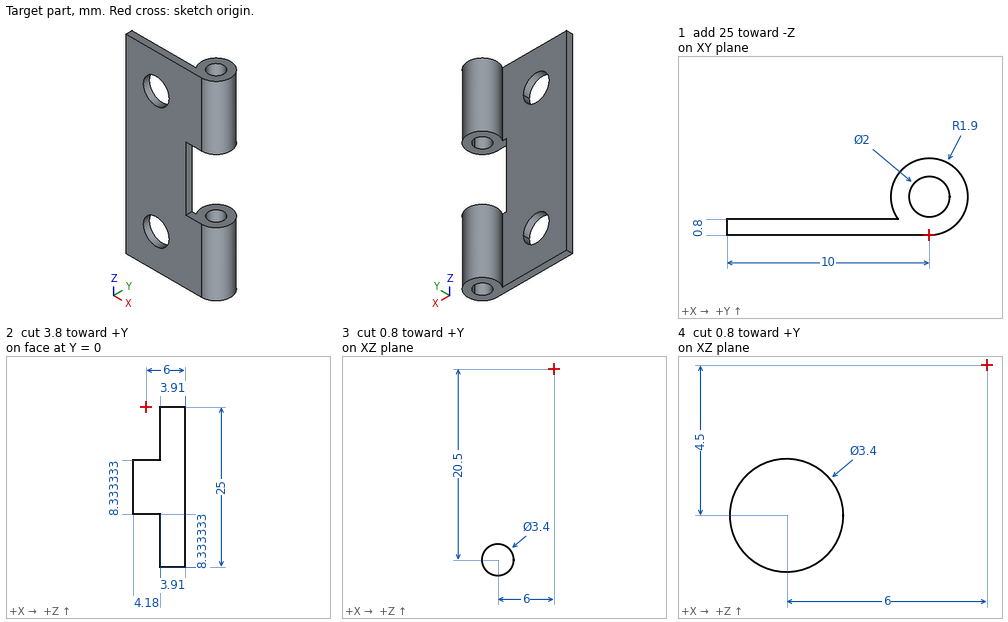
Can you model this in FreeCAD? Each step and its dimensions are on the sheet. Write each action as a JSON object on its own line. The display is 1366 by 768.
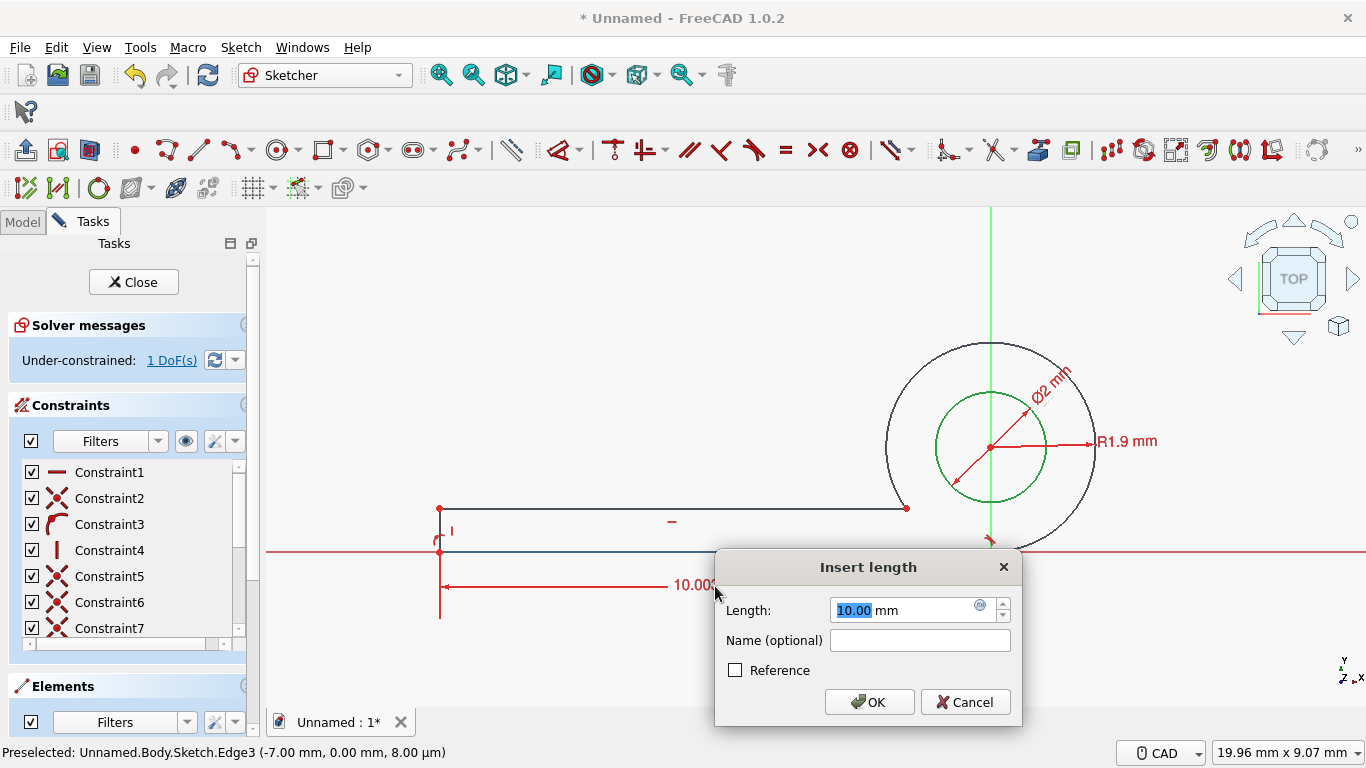
{"action": "type", "text": "10"}
{"action": "key", "text": "Return"}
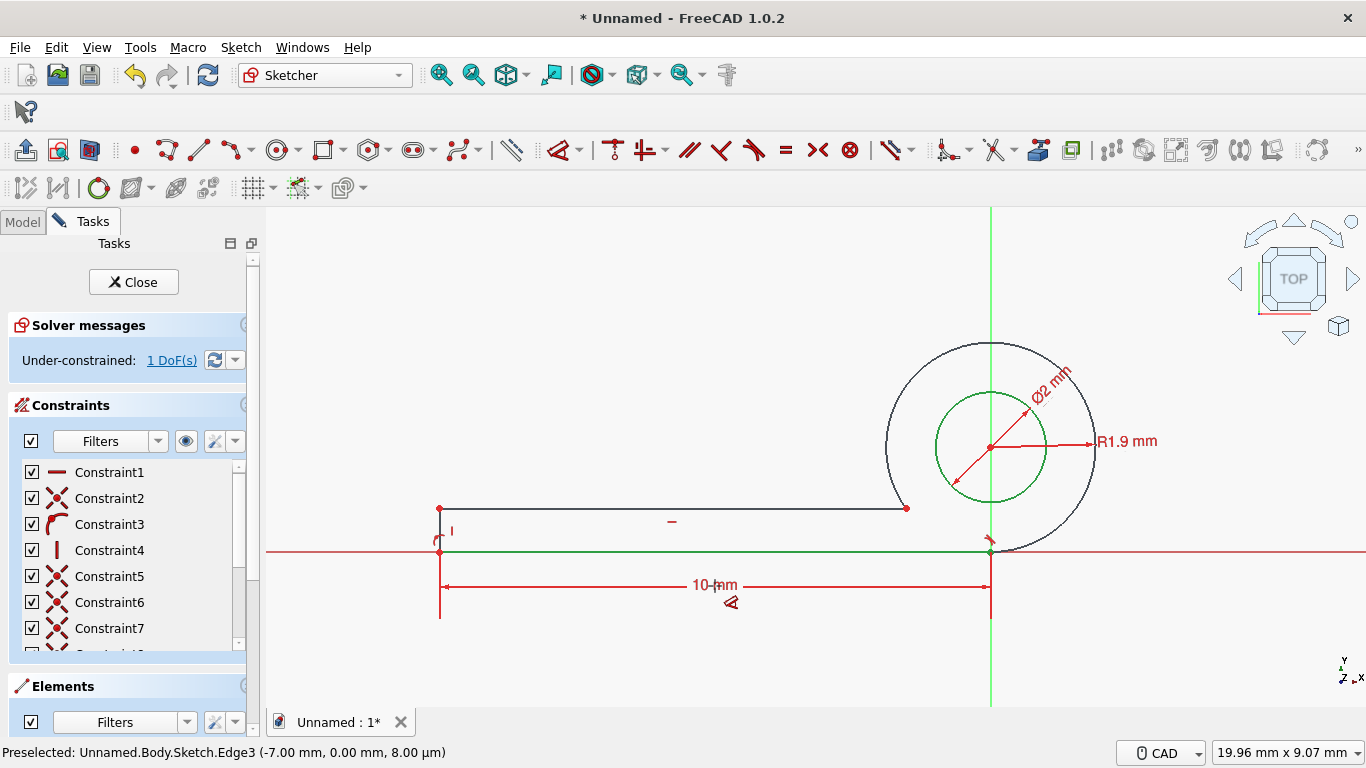
{"action": "left_click", "coordinate": [440, 522]}
{"action": "left_click", "coordinate": [406, 530]}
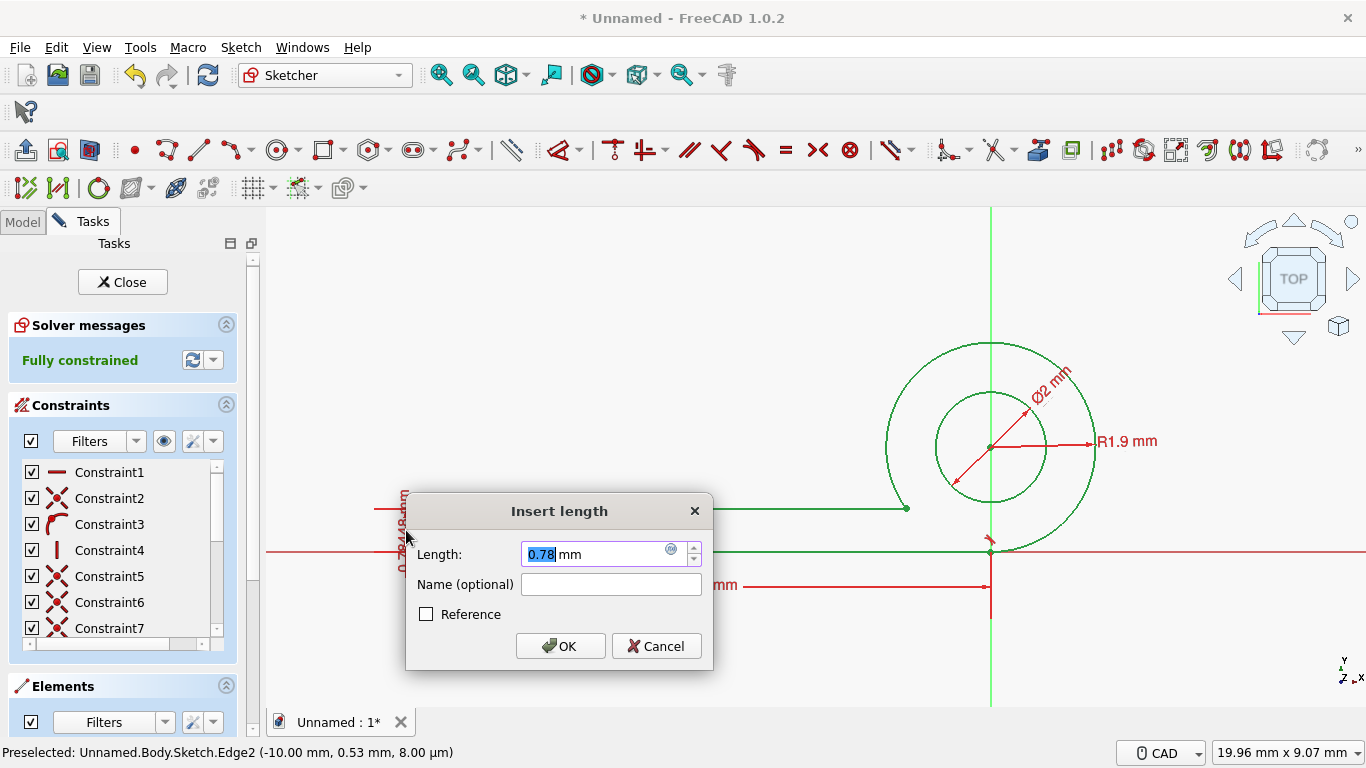
{"action": "type", "text": "0.8"}
{"action": "key", "text": "Return"}
{"action": "key", "text": "Escape"}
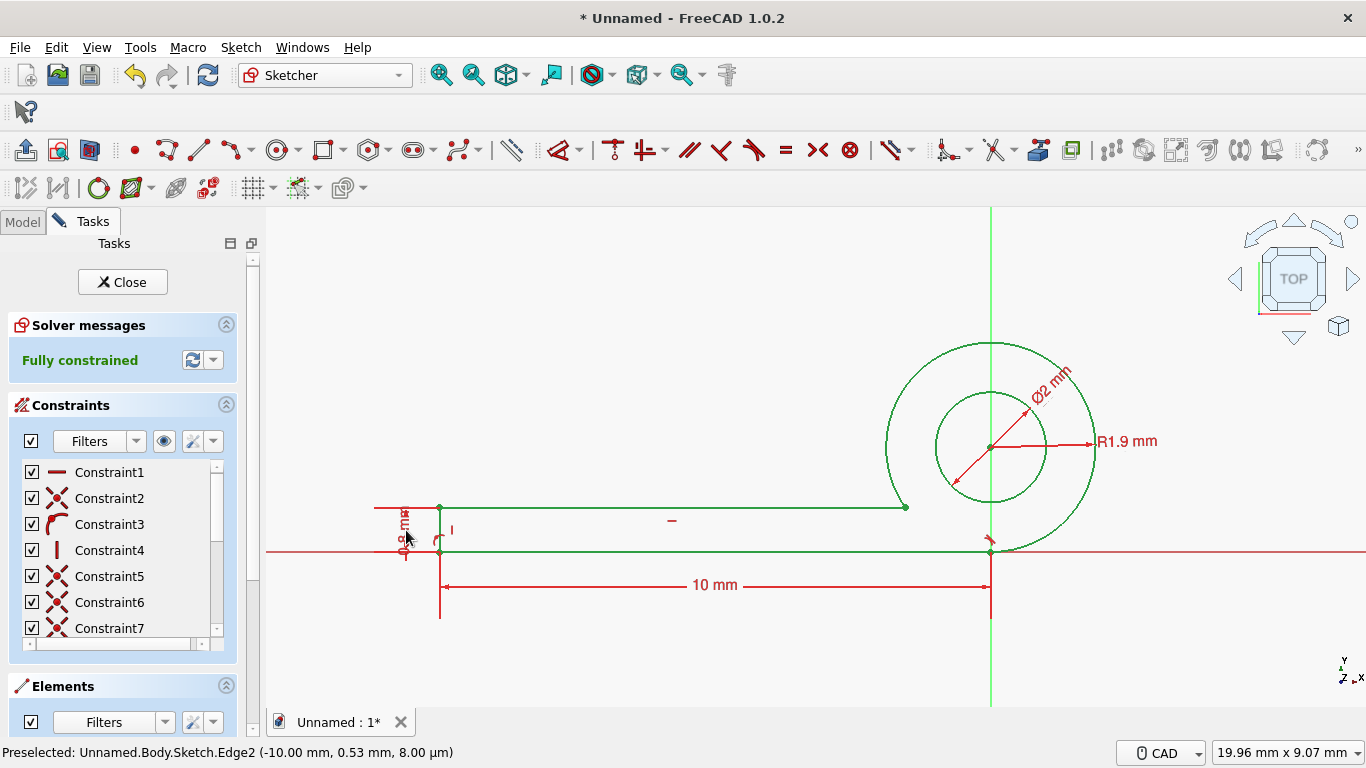
{"action": "left_click", "coordinate": [123, 282]}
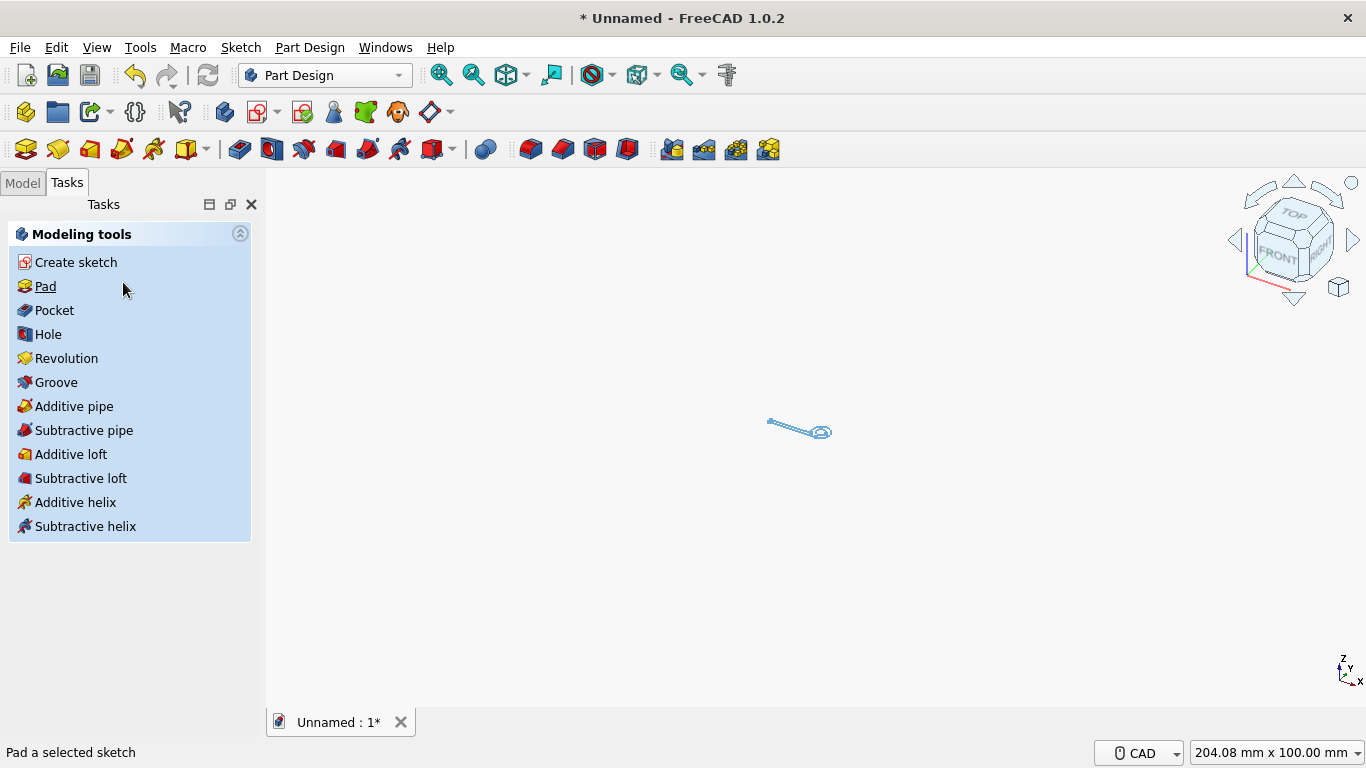
{"action": "left_click", "coordinate": [26, 150]}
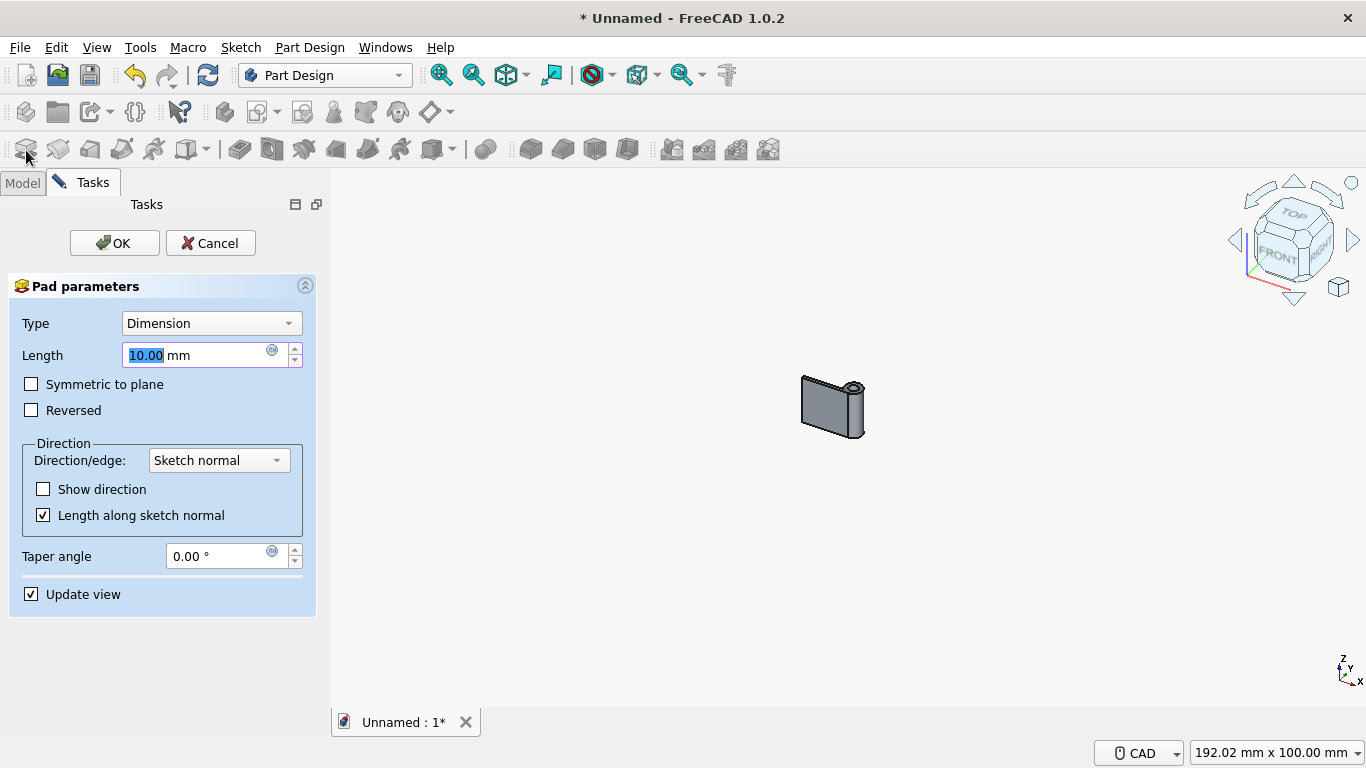
{"action": "type", "text": "25"}
{"action": "key", "text": "Tab"}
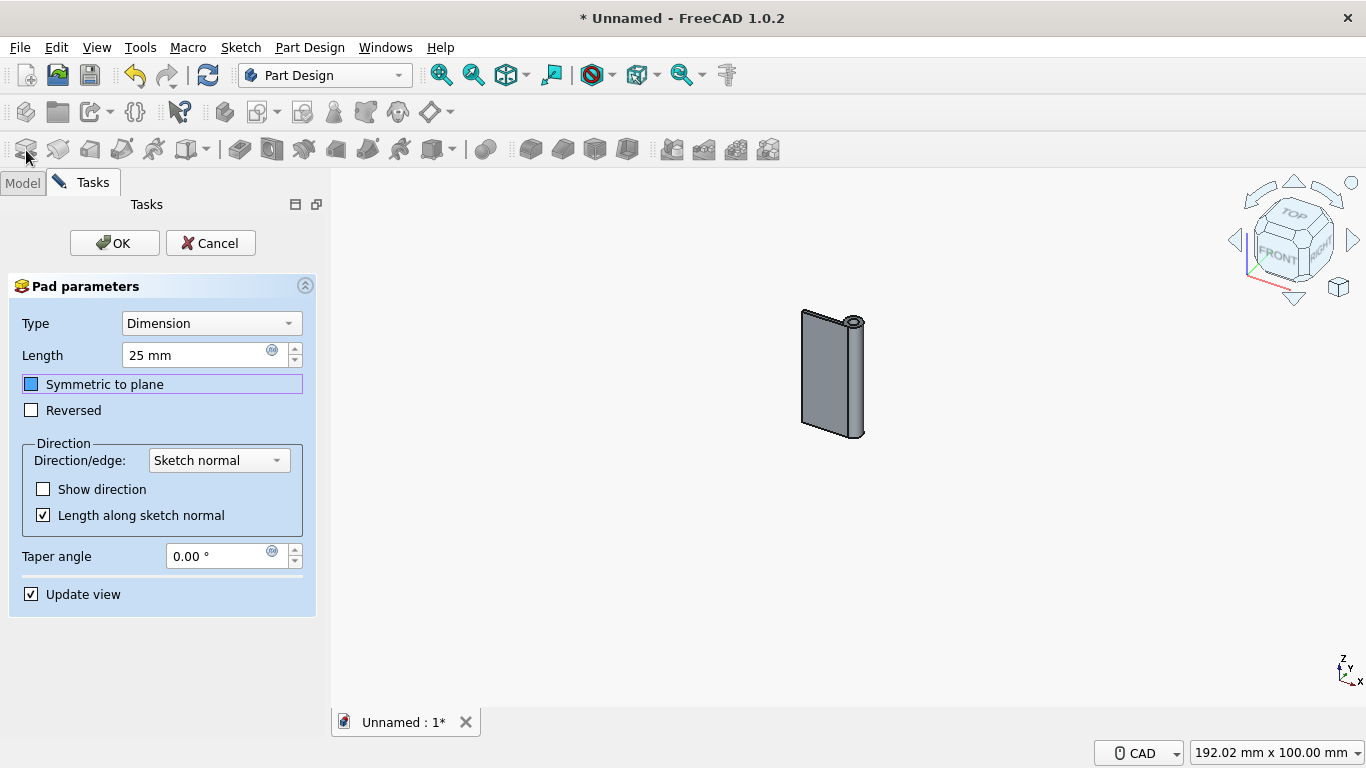
{"action": "left_click", "coordinate": [30, 410]}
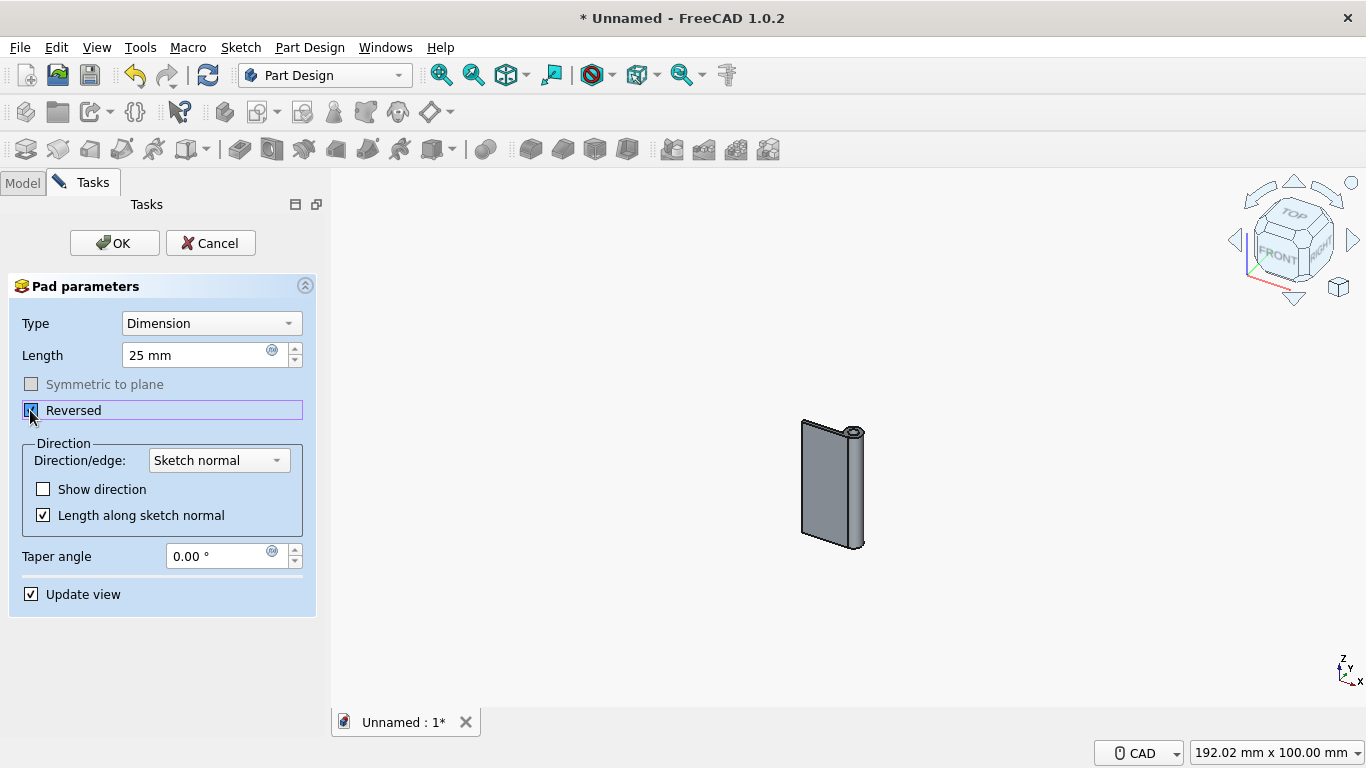
{"action": "left_click", "coordinate": [115, 243]}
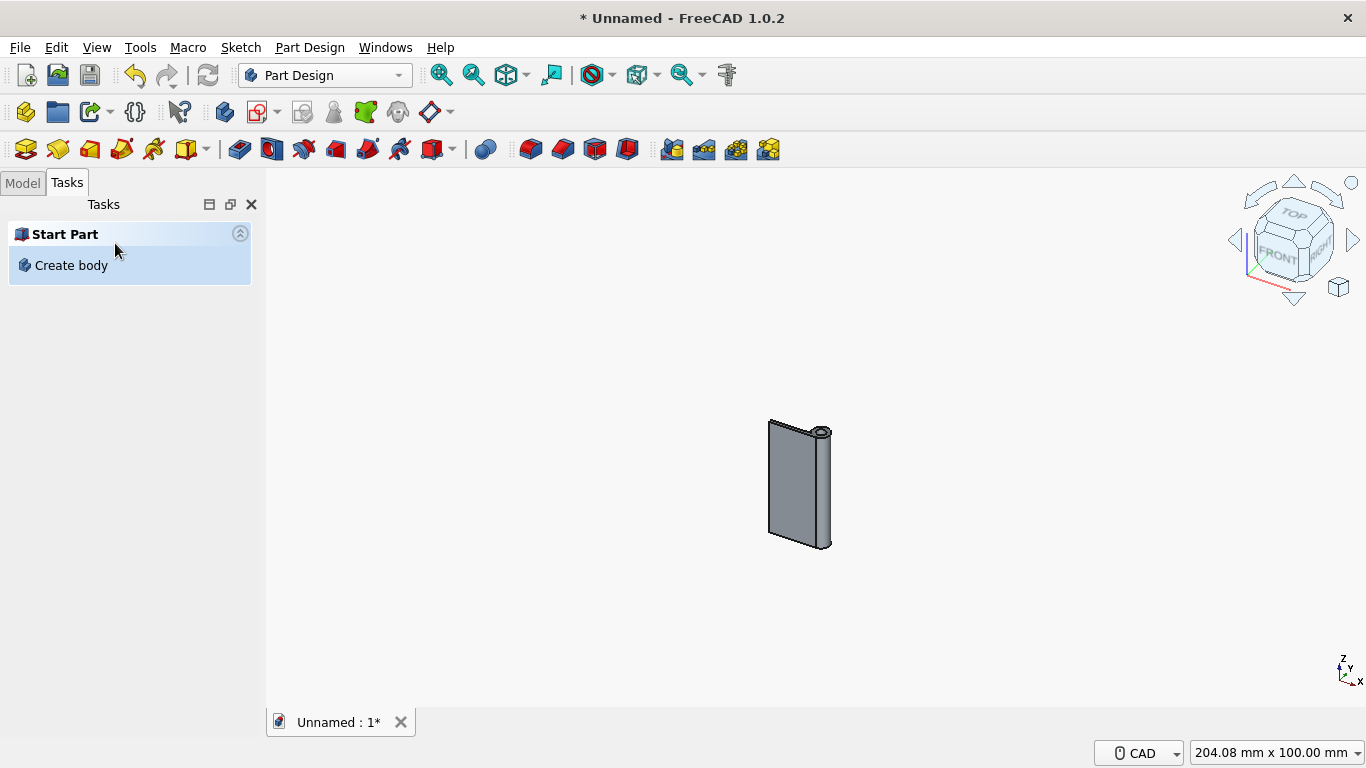
{"action": "left_click", "coordinate": [442, 76]}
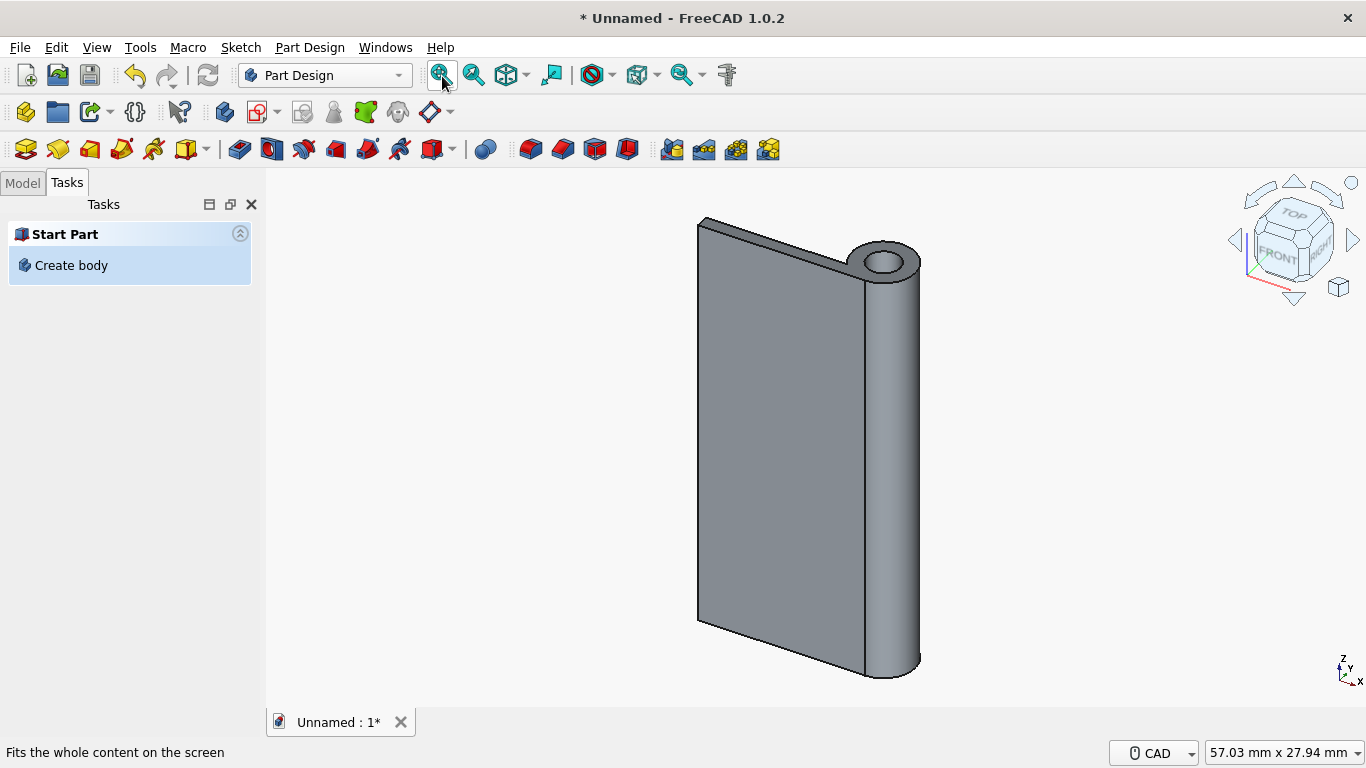
{"action": "left_click", "coordinate": [782, 337]}